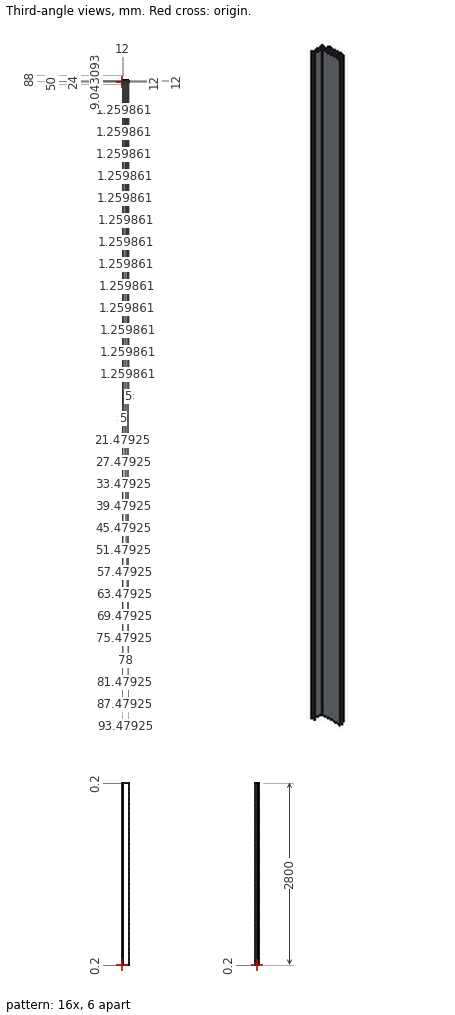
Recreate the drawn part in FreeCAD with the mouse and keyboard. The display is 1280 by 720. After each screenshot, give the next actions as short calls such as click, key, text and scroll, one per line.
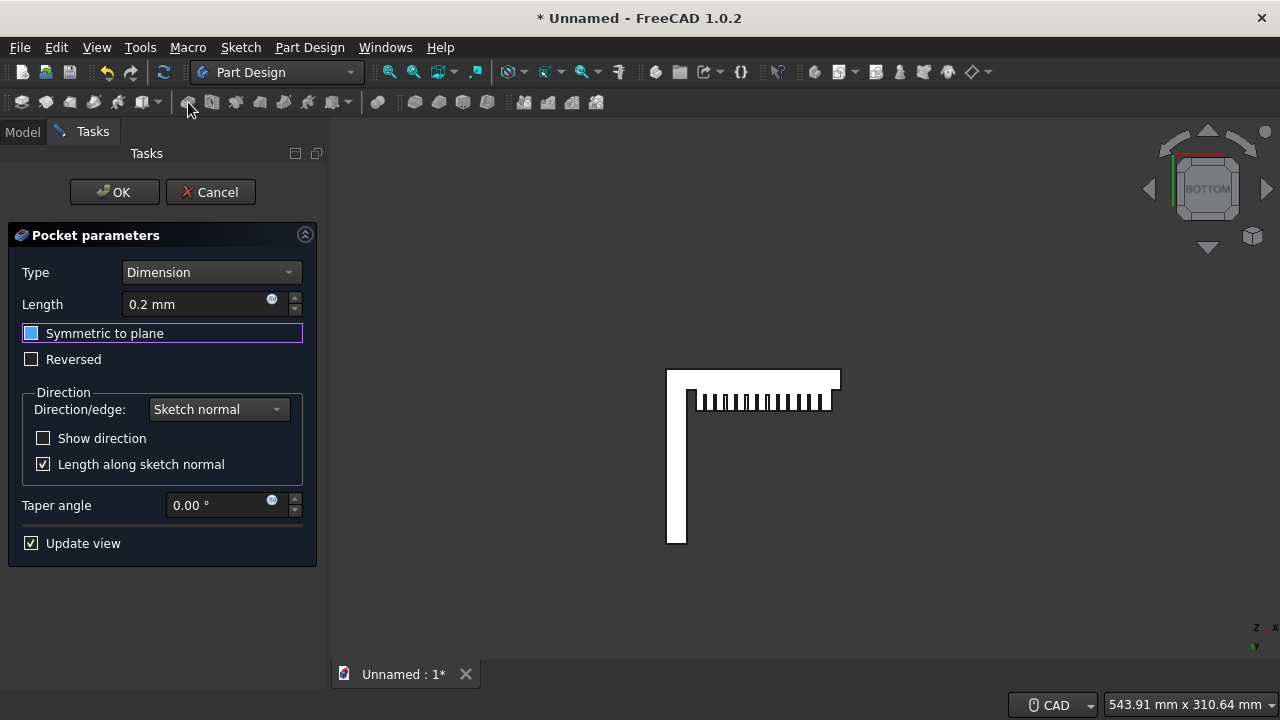
click(115, 192)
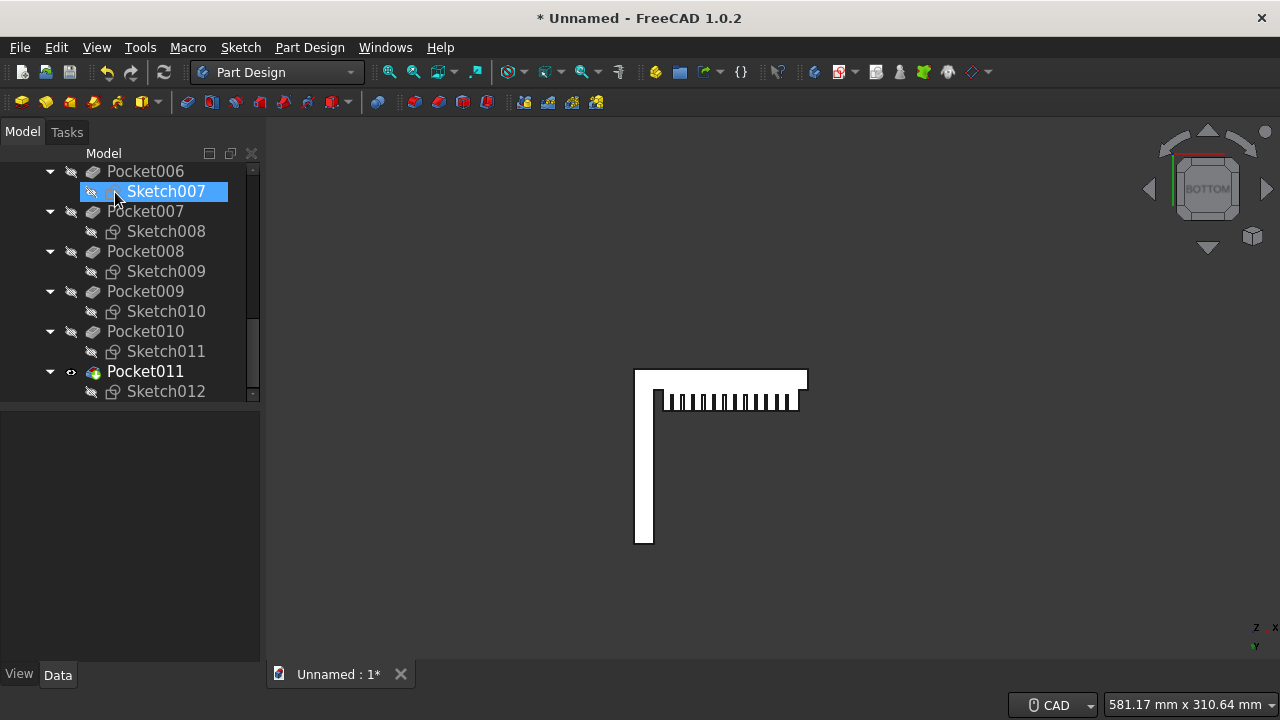
click(390, 72)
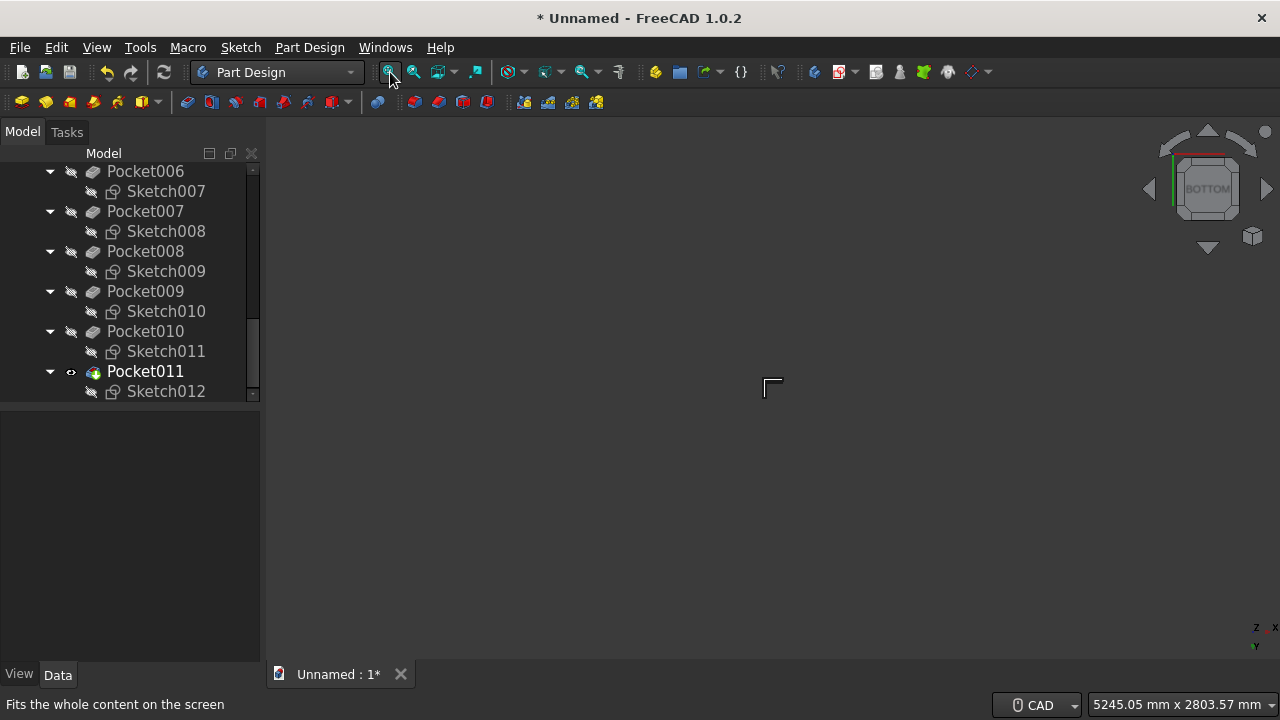
click(840, 72)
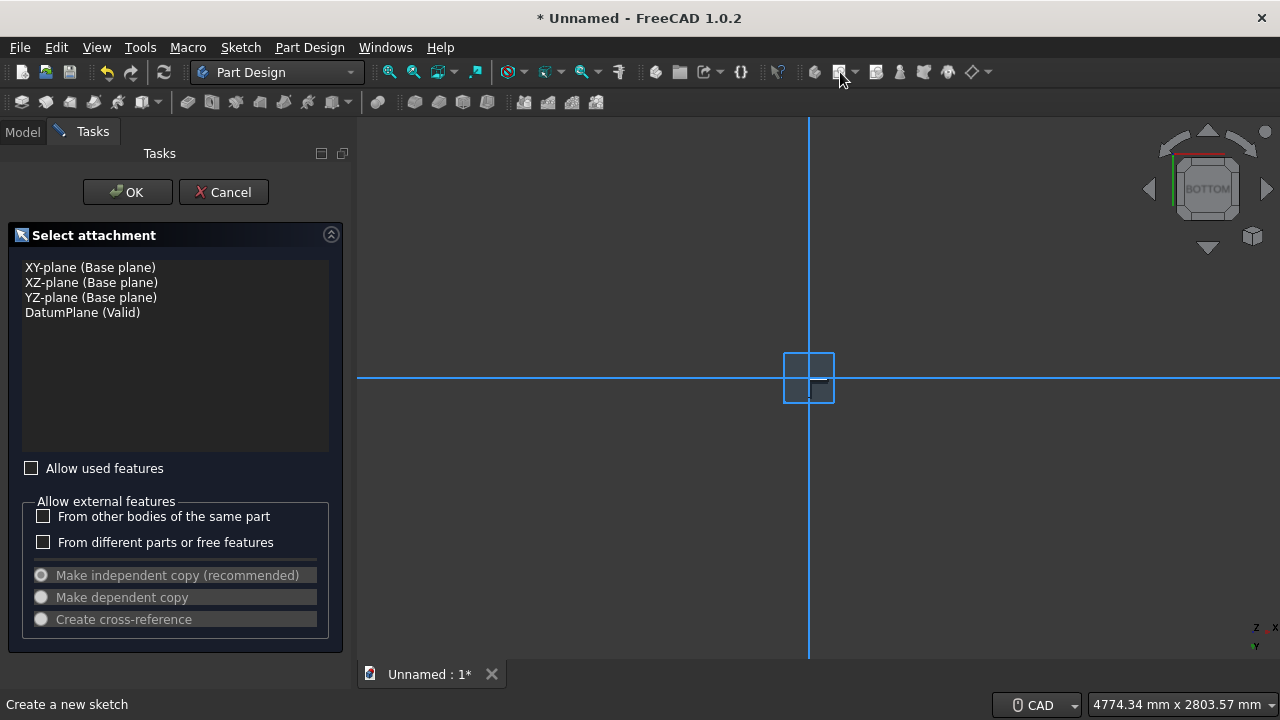
click(82, 268)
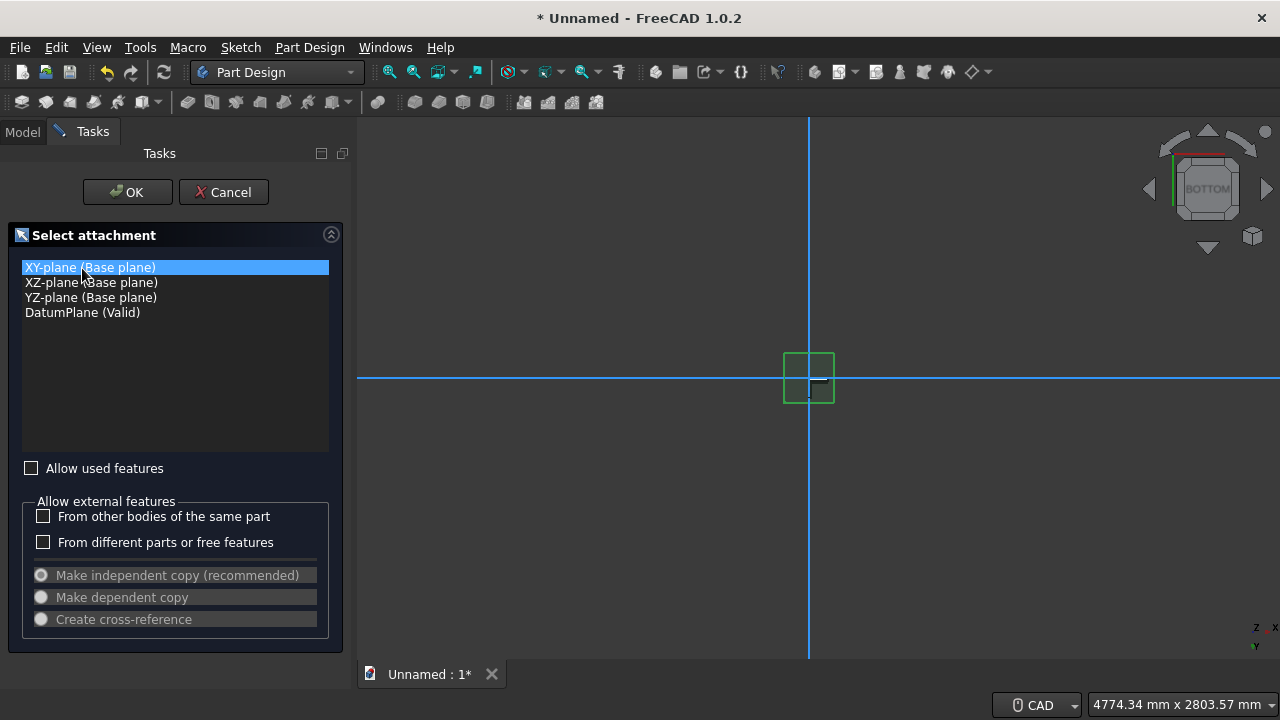
click(128, 192)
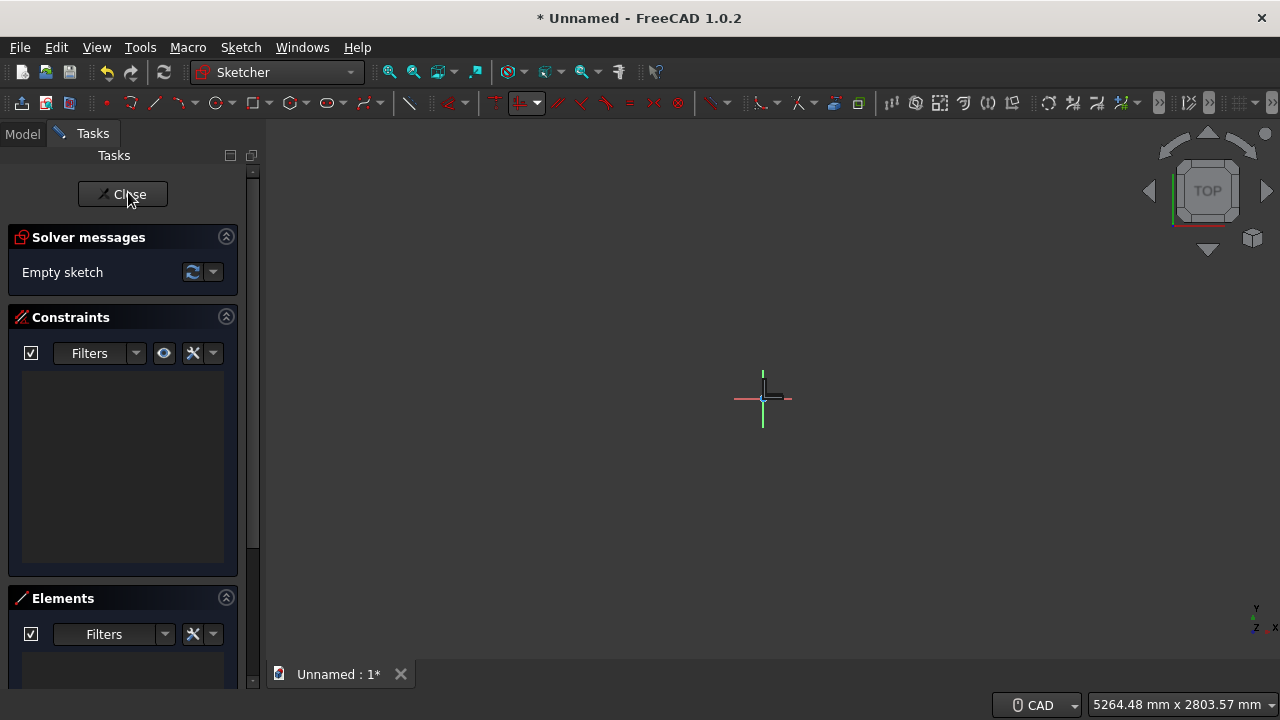
click(70, 104)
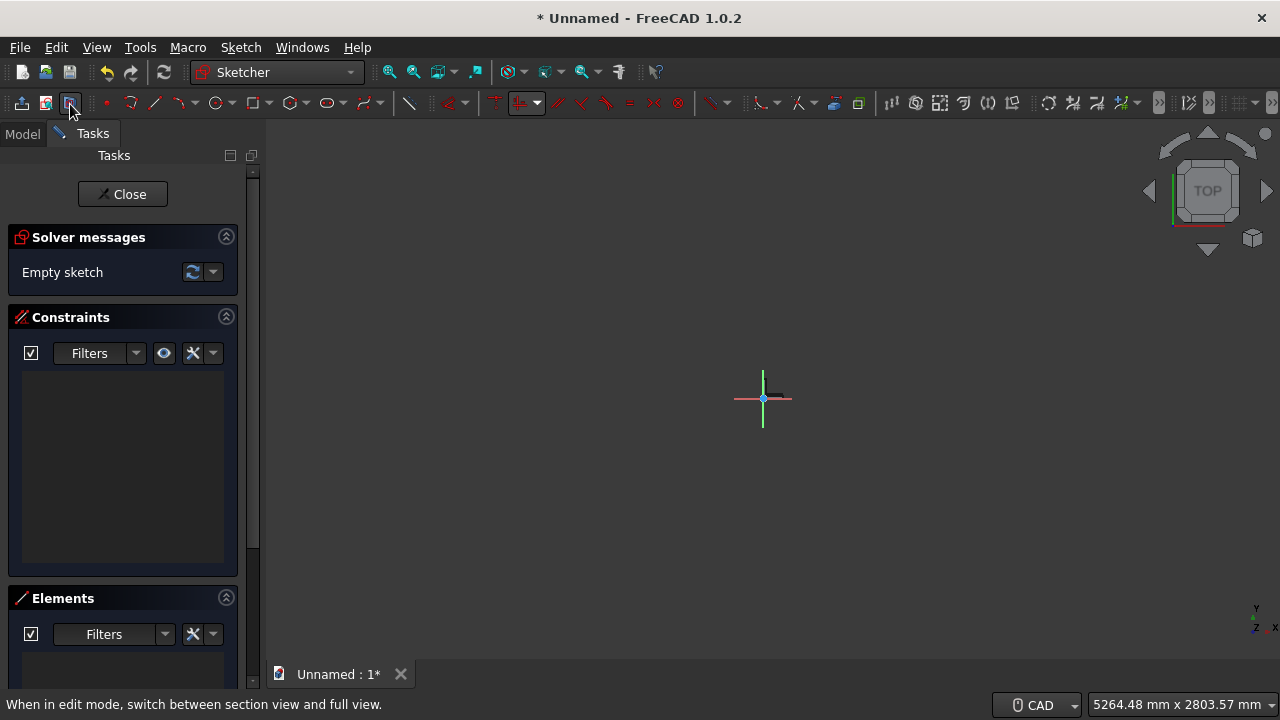
scroll(786, 395, up, 15)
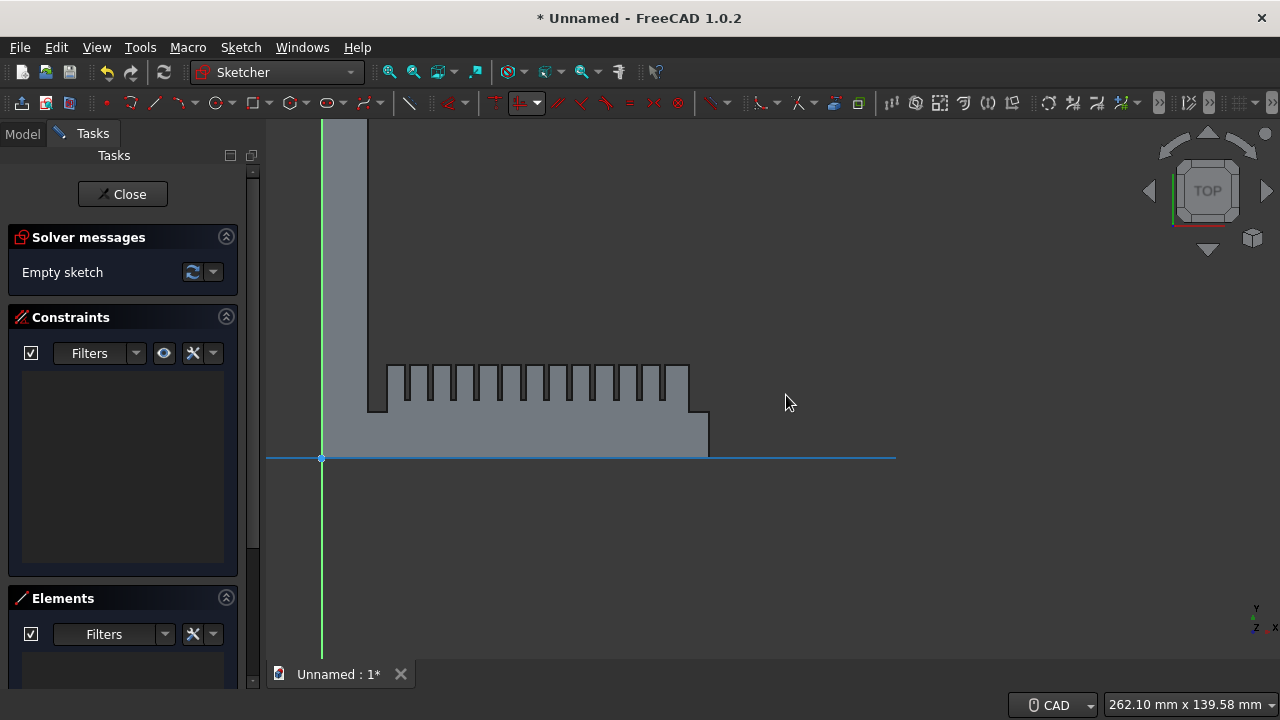
scroll(683, 382, up, 11)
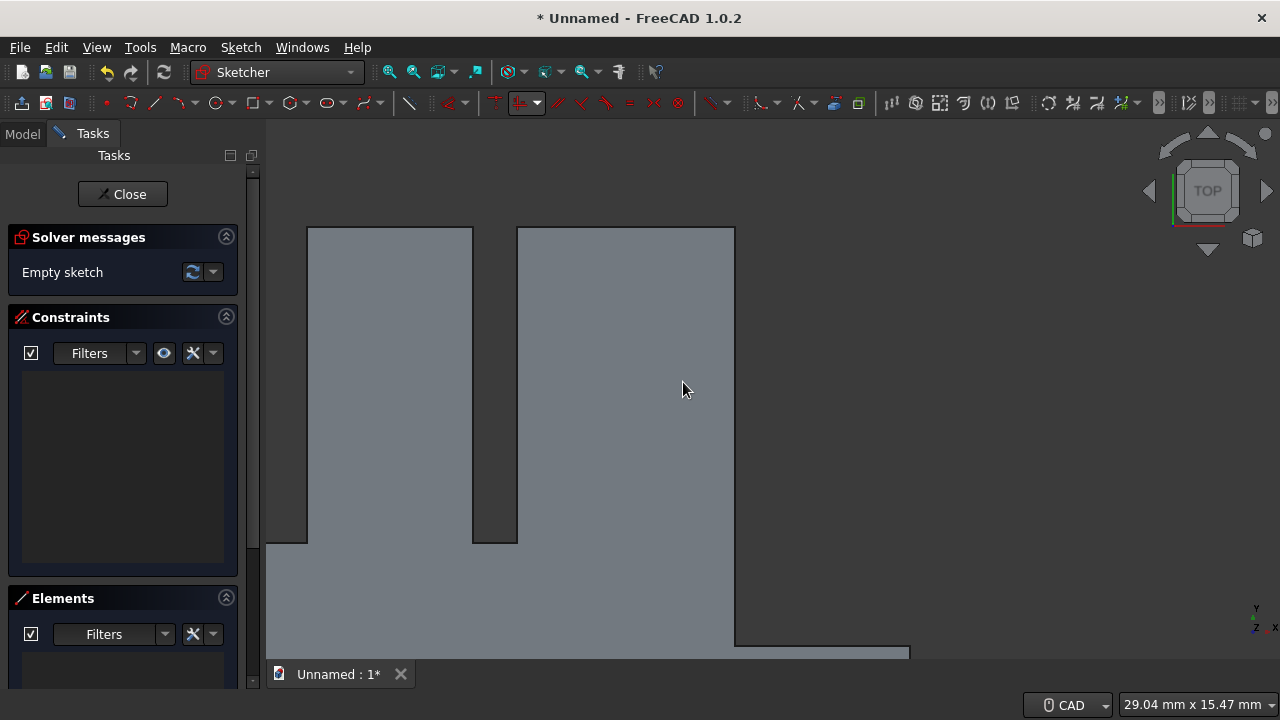
click(254, 104)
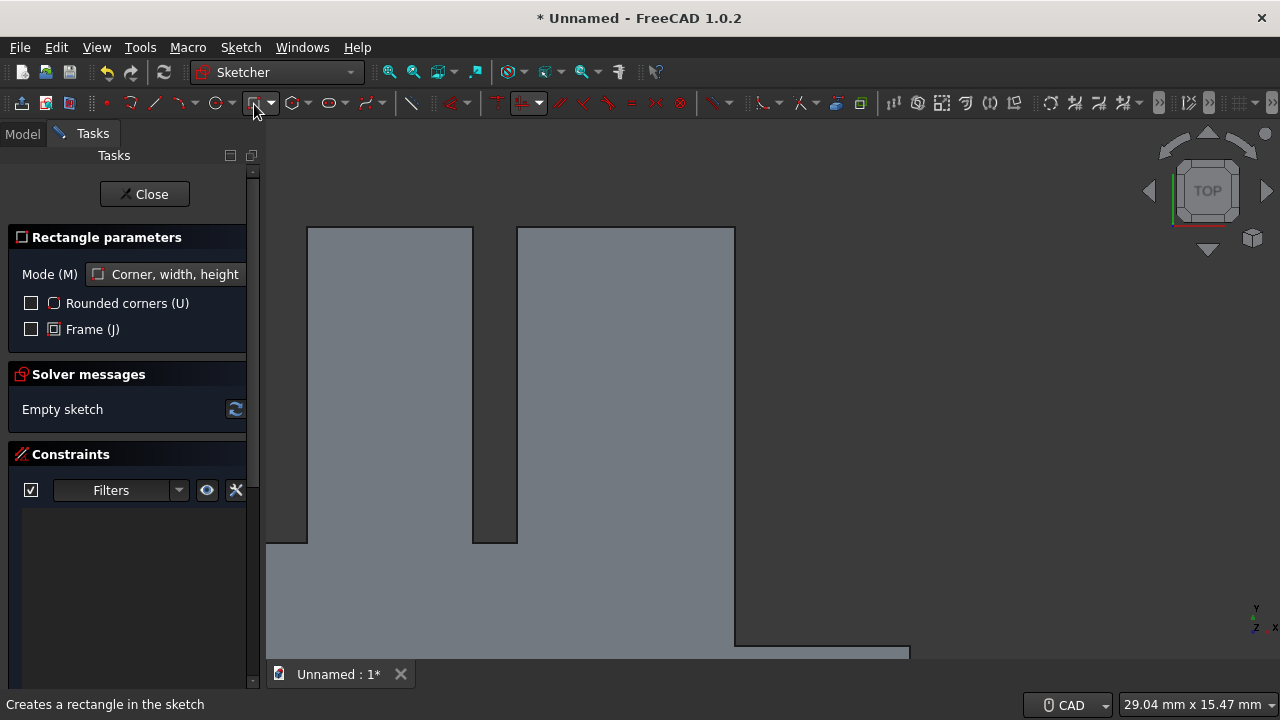
click(682, 227)
move(726, 543)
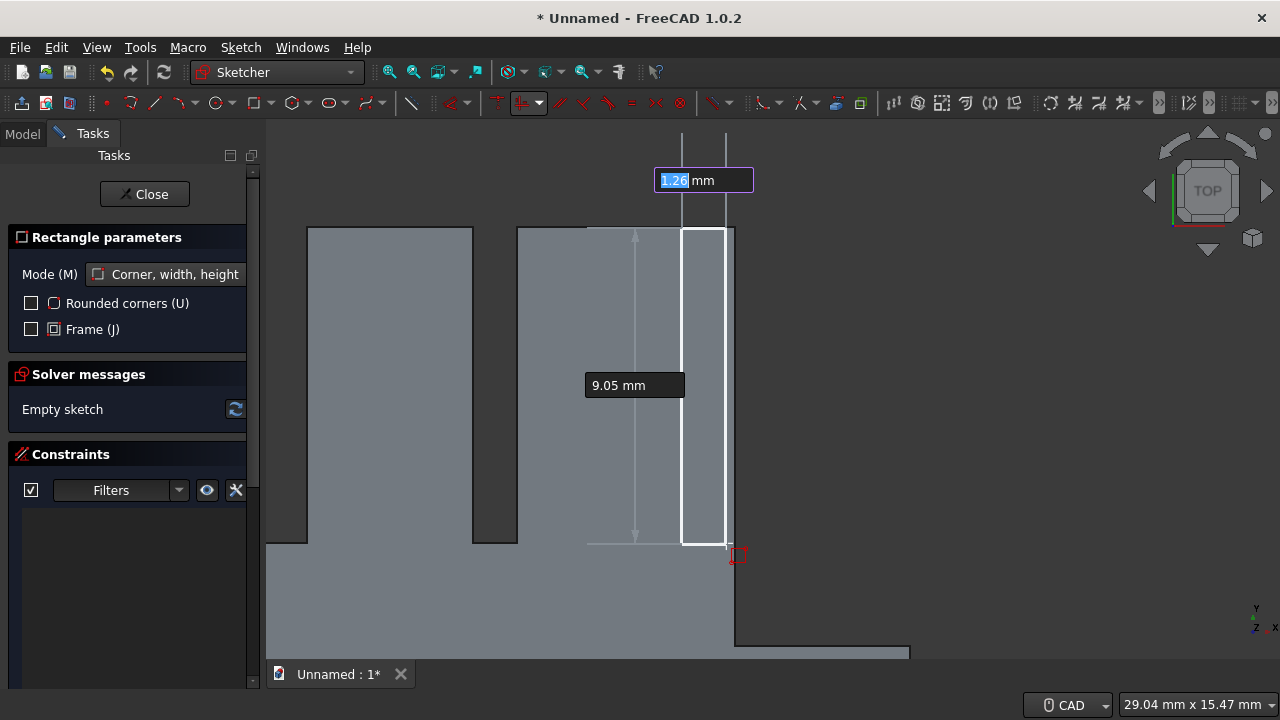
text(1.259861)
key(Tab)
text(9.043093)
key(Return)
key(Escape)